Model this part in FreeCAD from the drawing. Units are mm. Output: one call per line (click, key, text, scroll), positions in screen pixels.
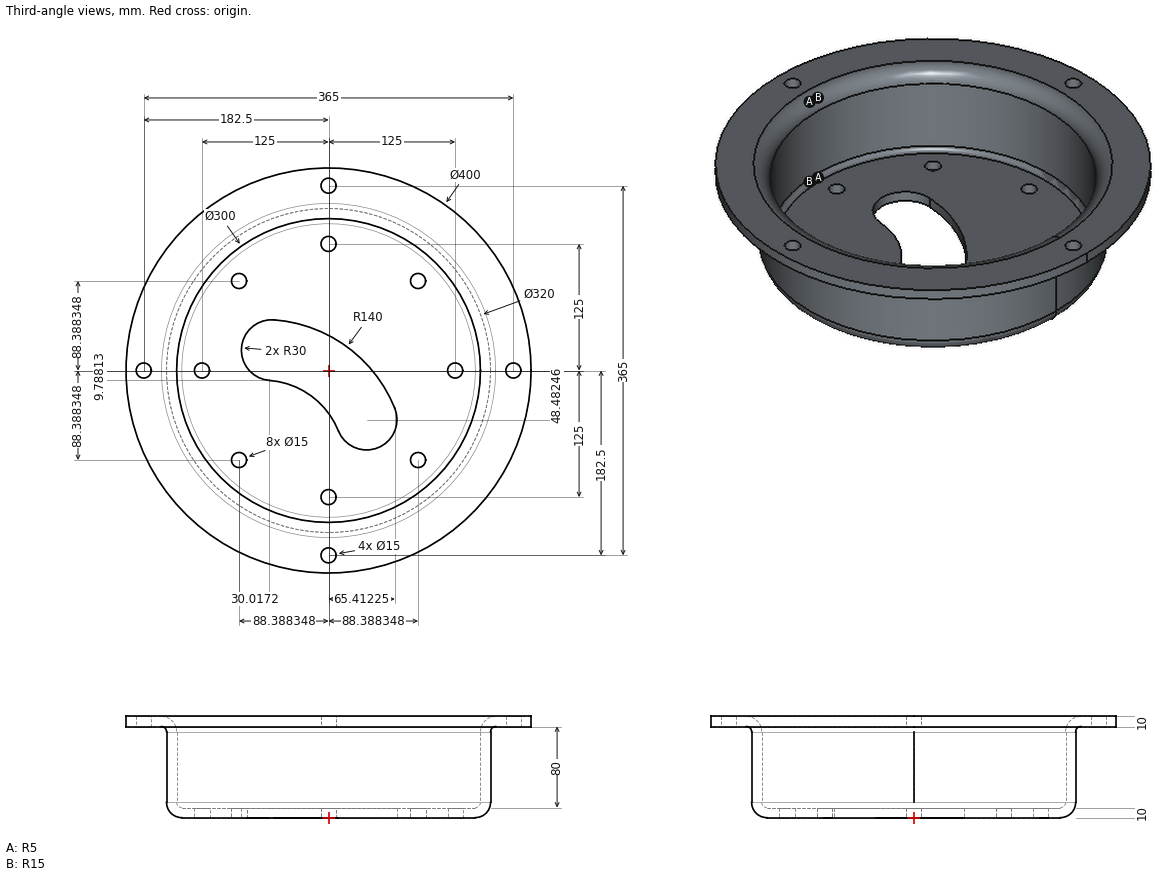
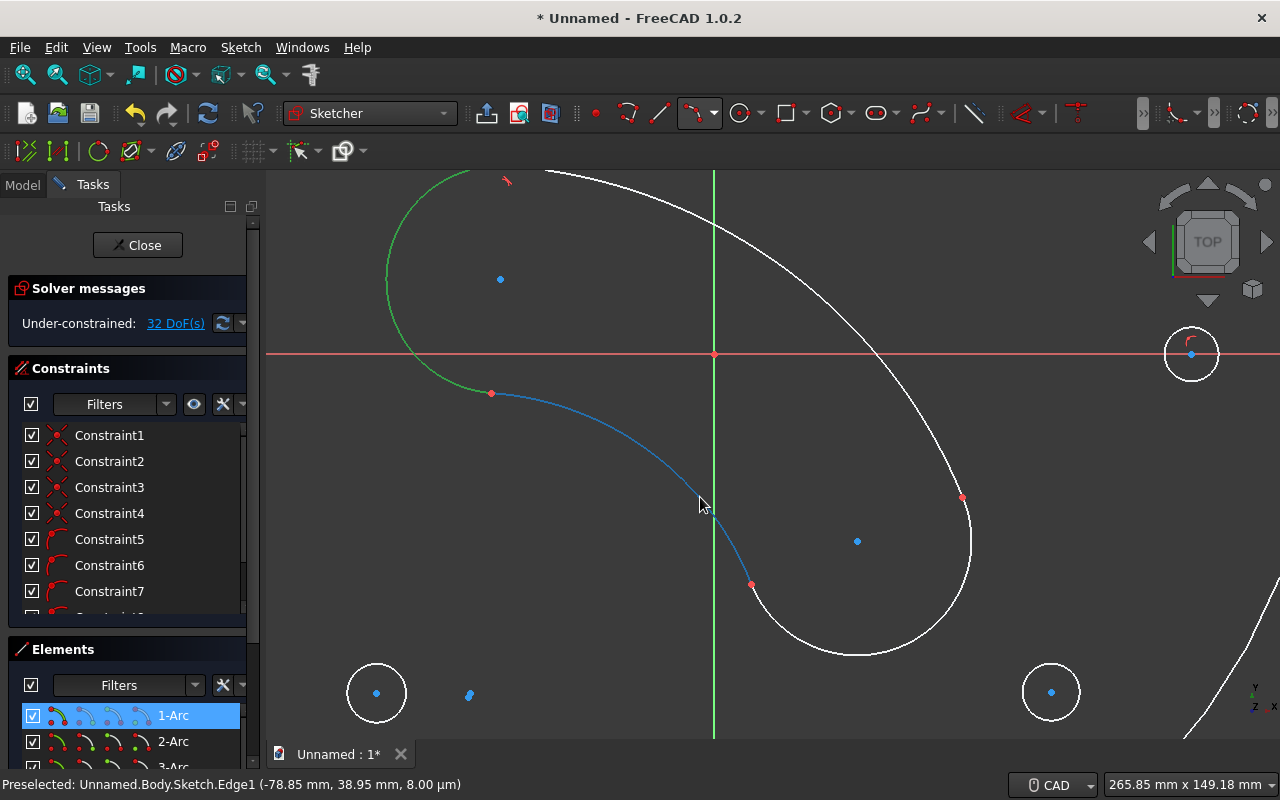
click(699, 497)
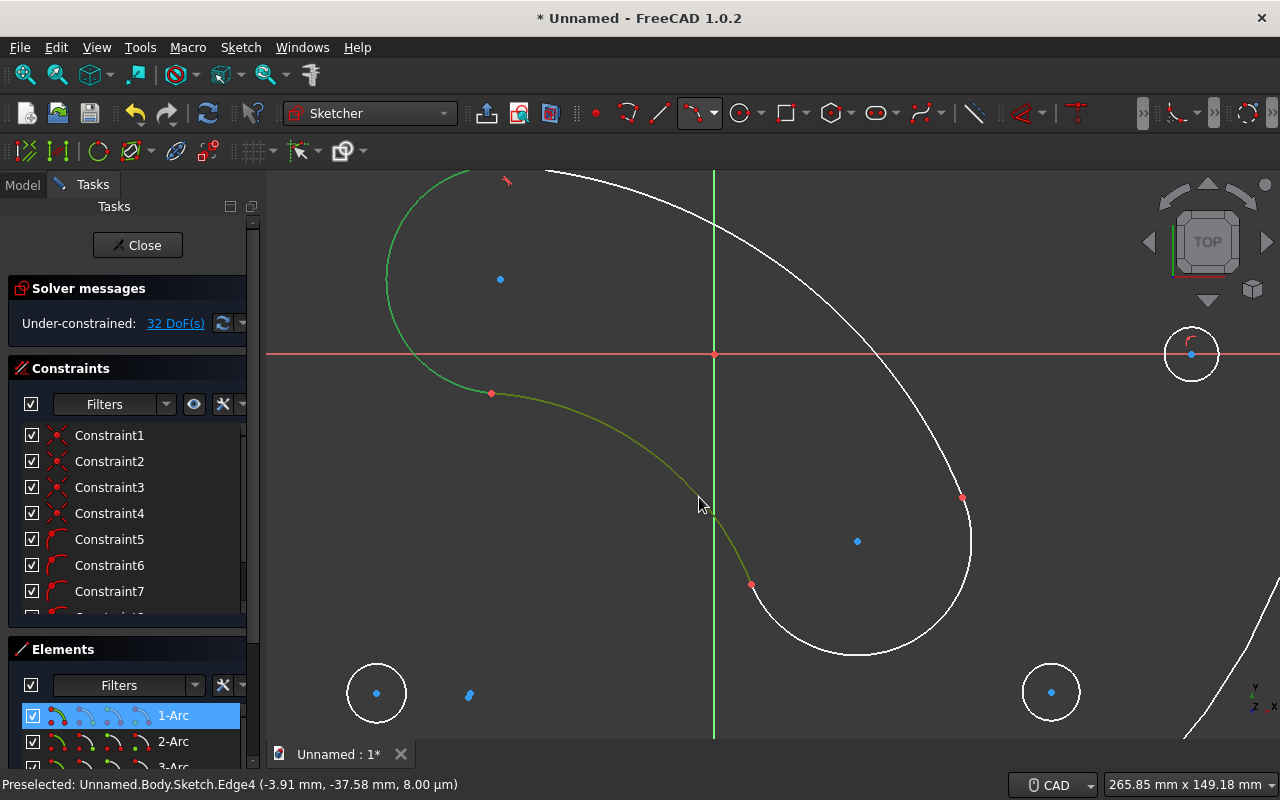
key(t)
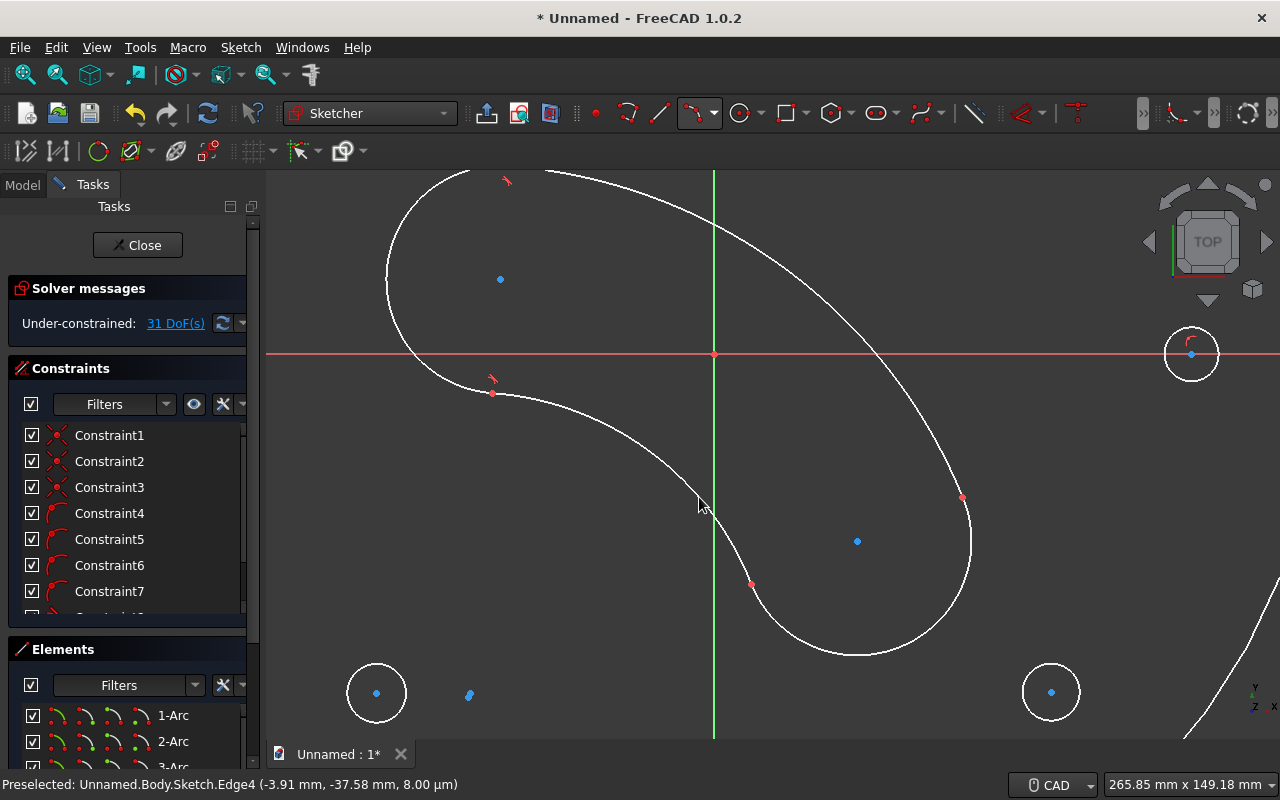
click(681, 208)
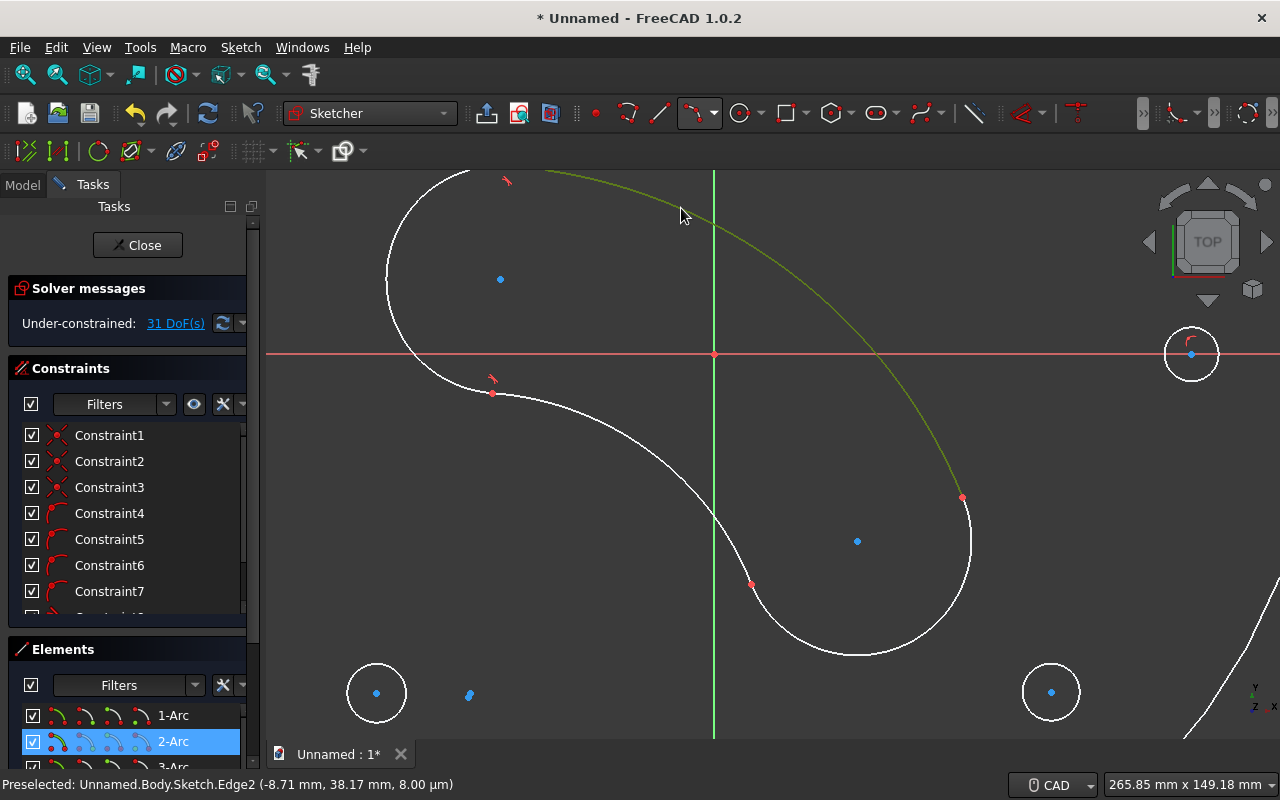
click(830, 652)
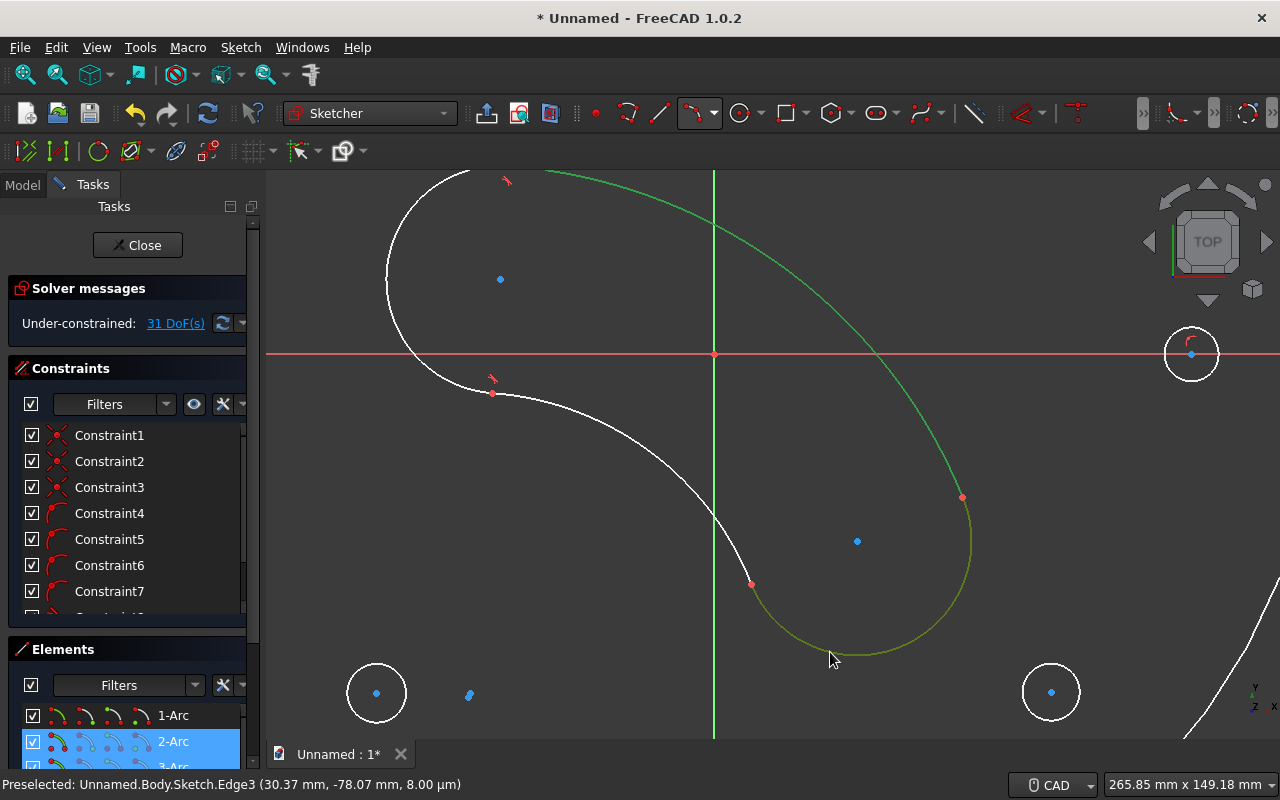
key(t)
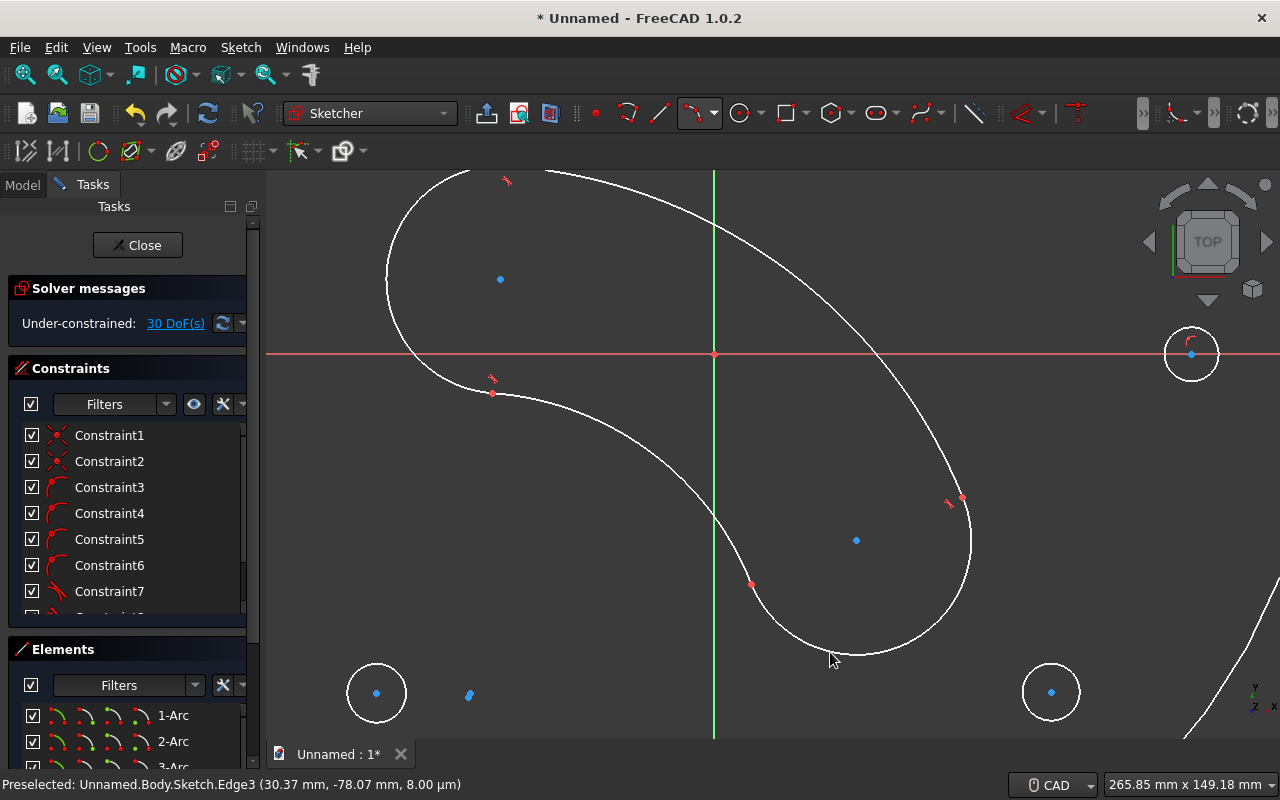
click(830, 652)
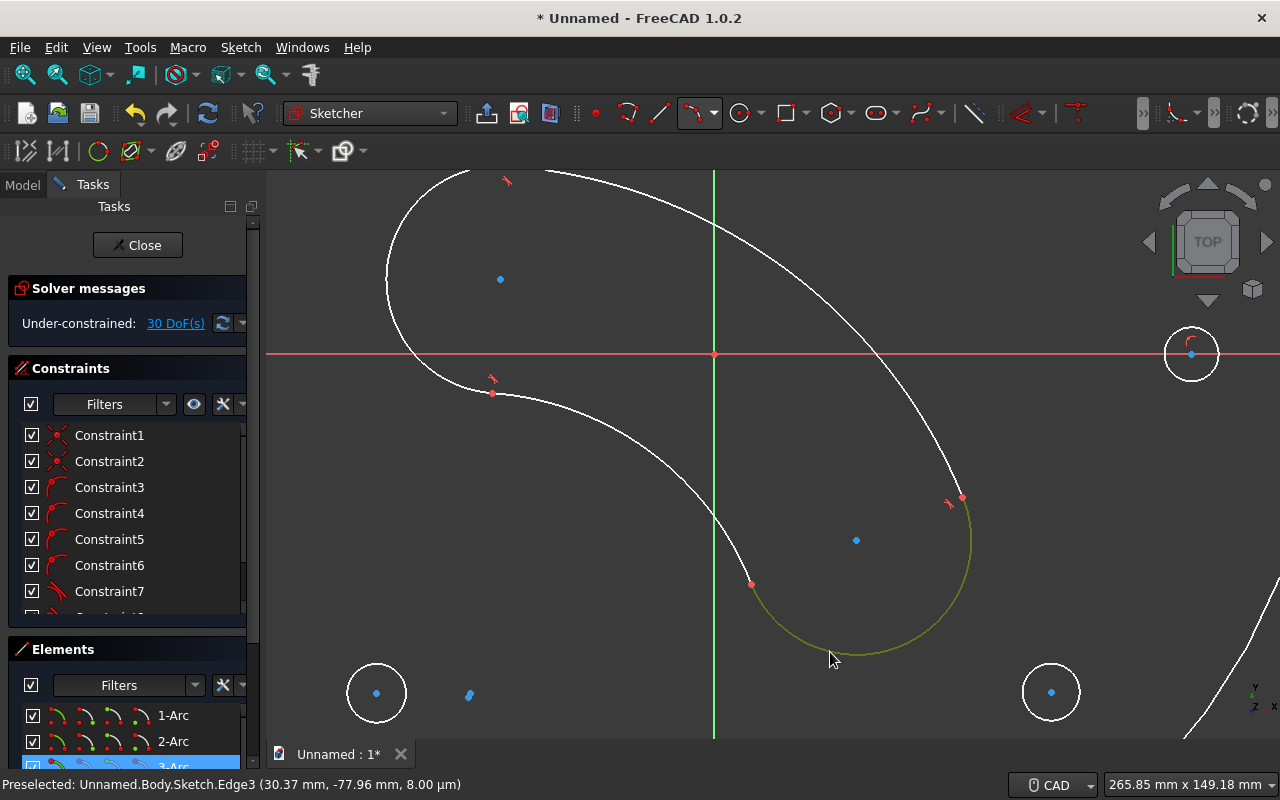
click(699, 497)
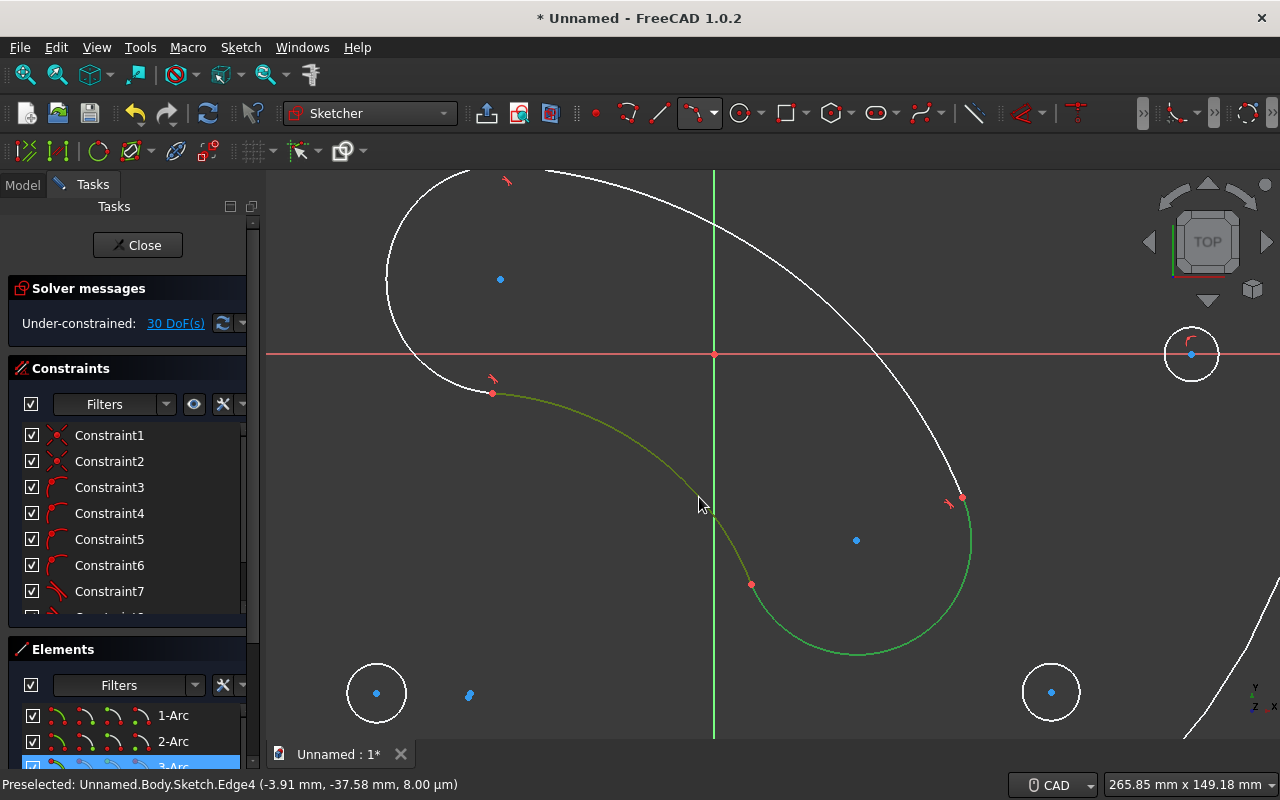
key(t)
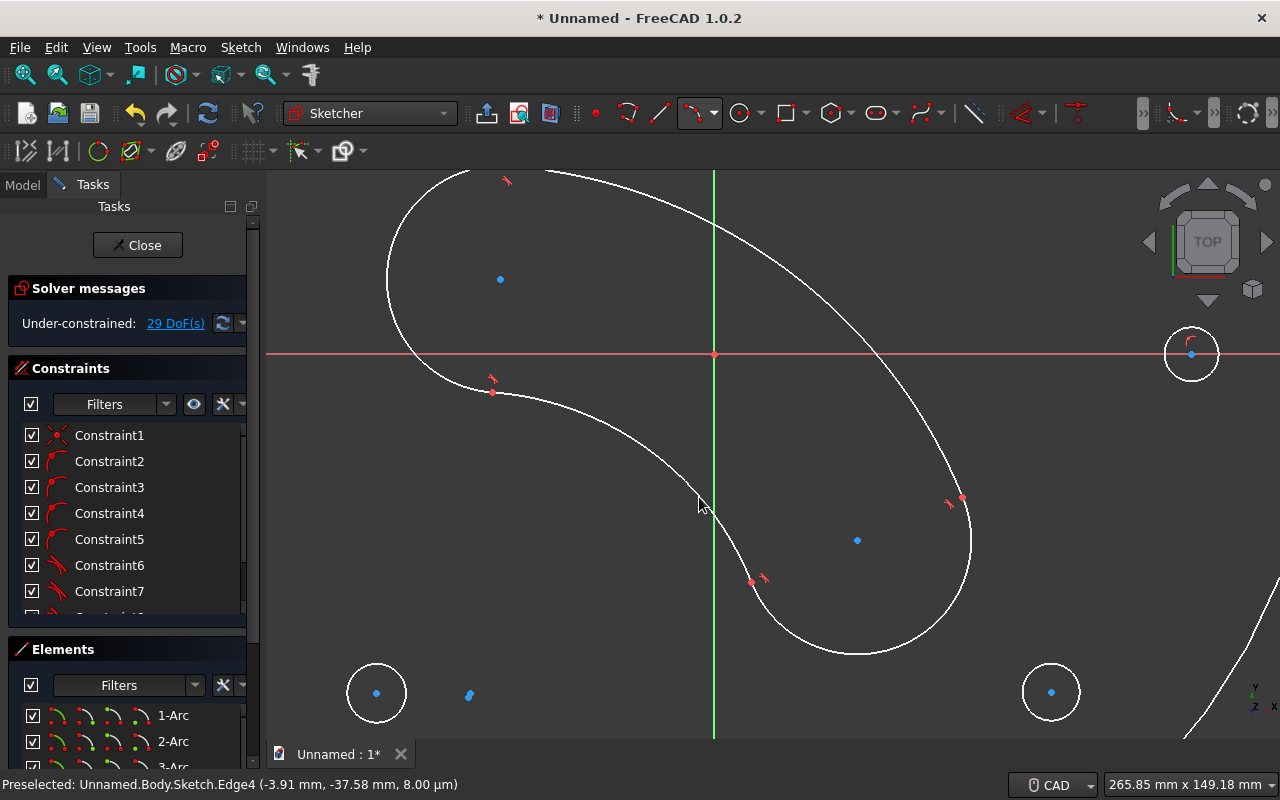
click(681, 208)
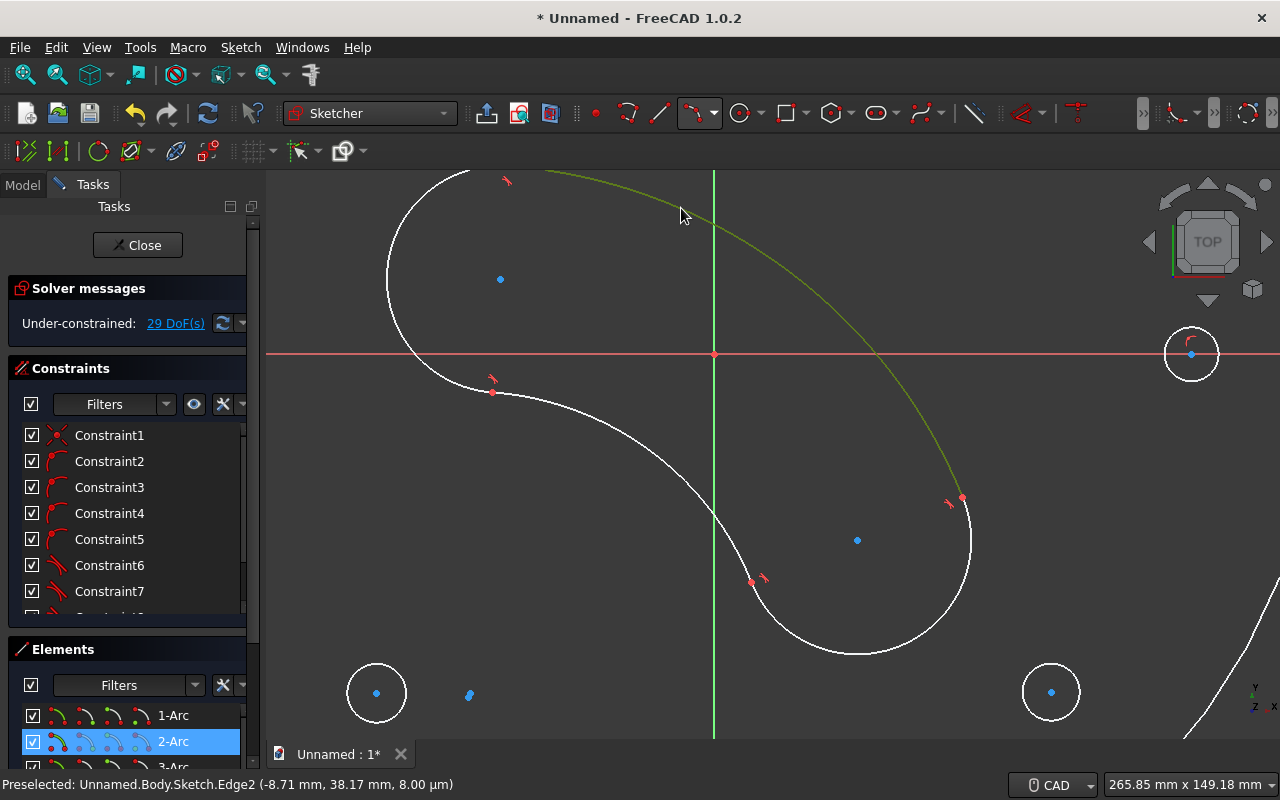
click(699, 496)